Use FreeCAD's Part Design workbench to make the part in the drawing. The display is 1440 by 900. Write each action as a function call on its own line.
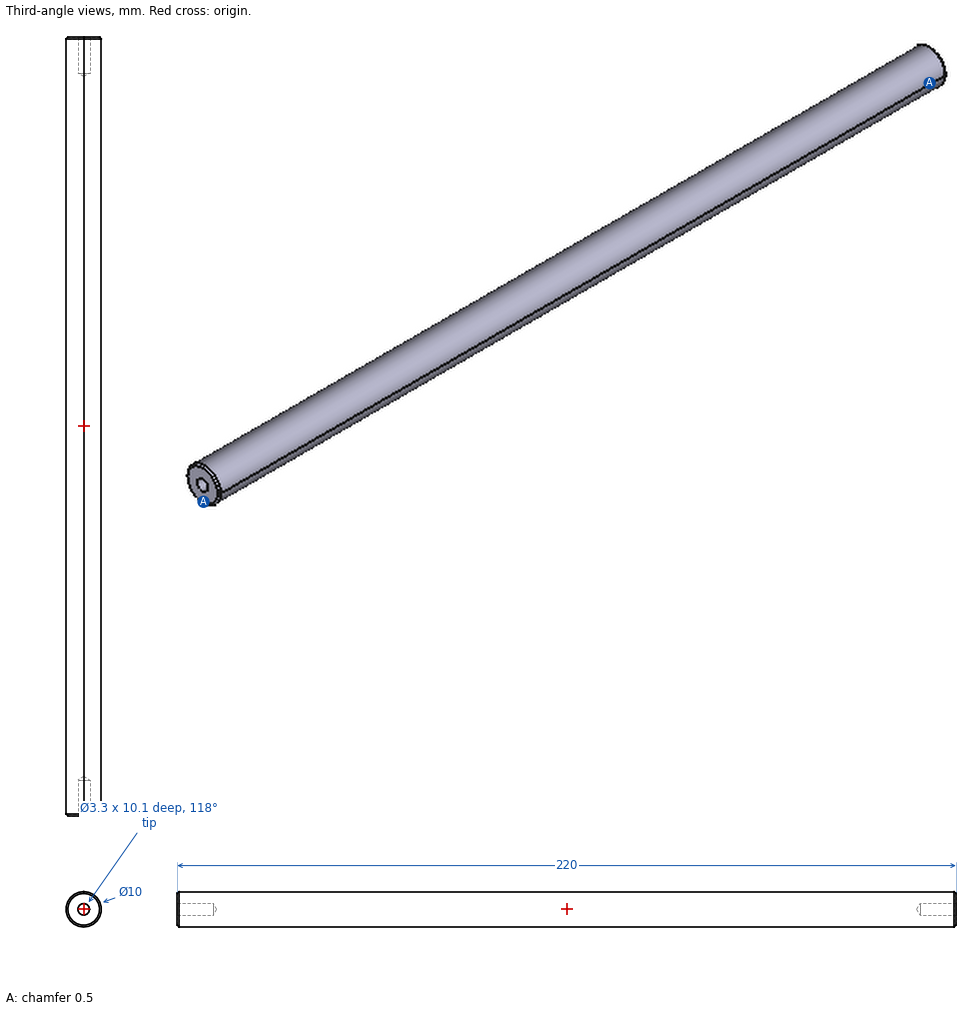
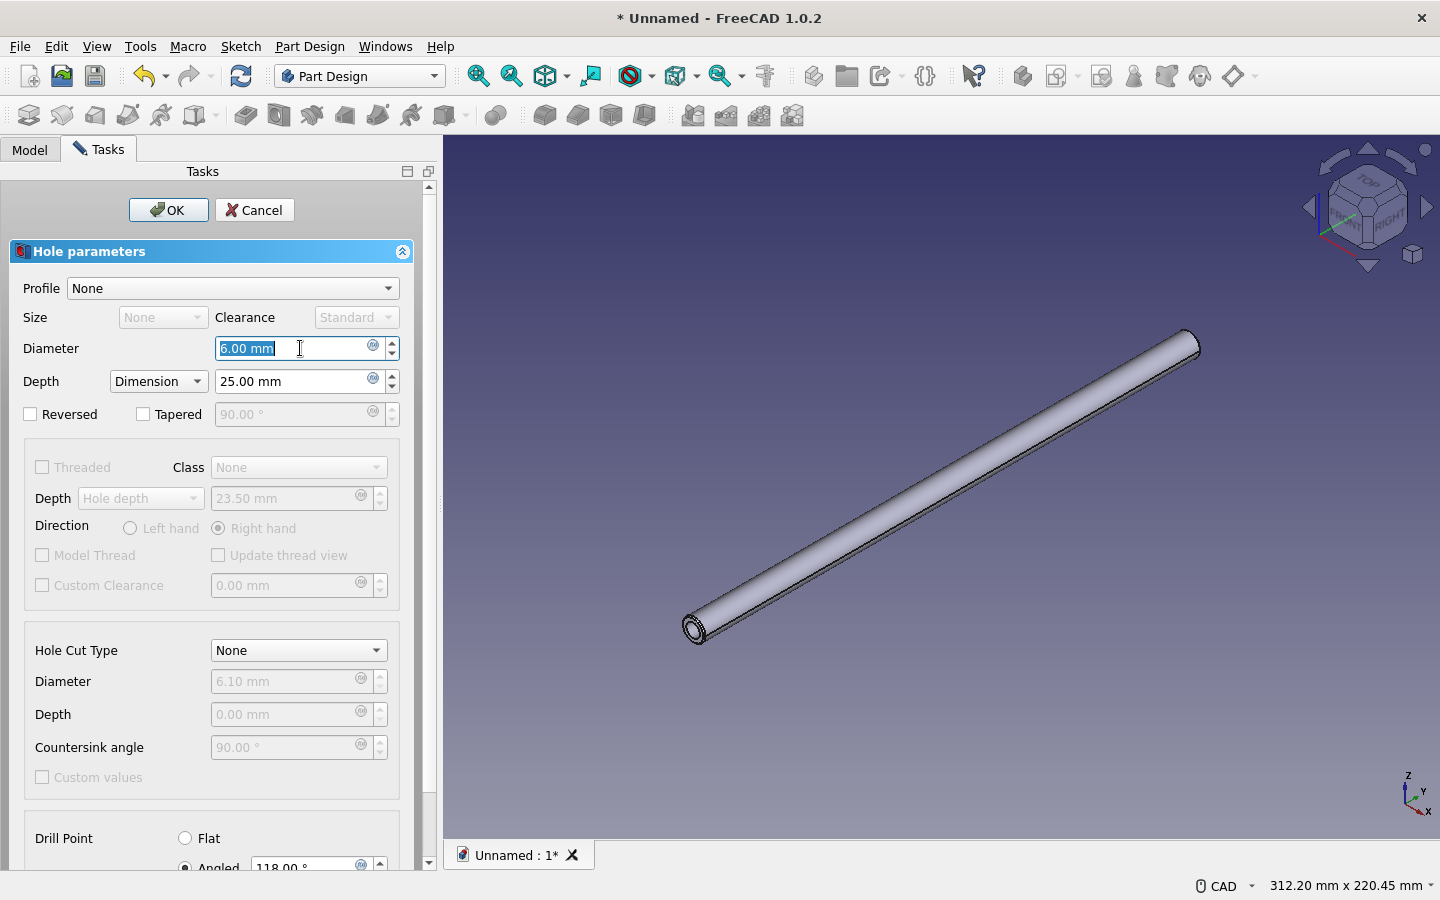
text(3.3)
key(Tab)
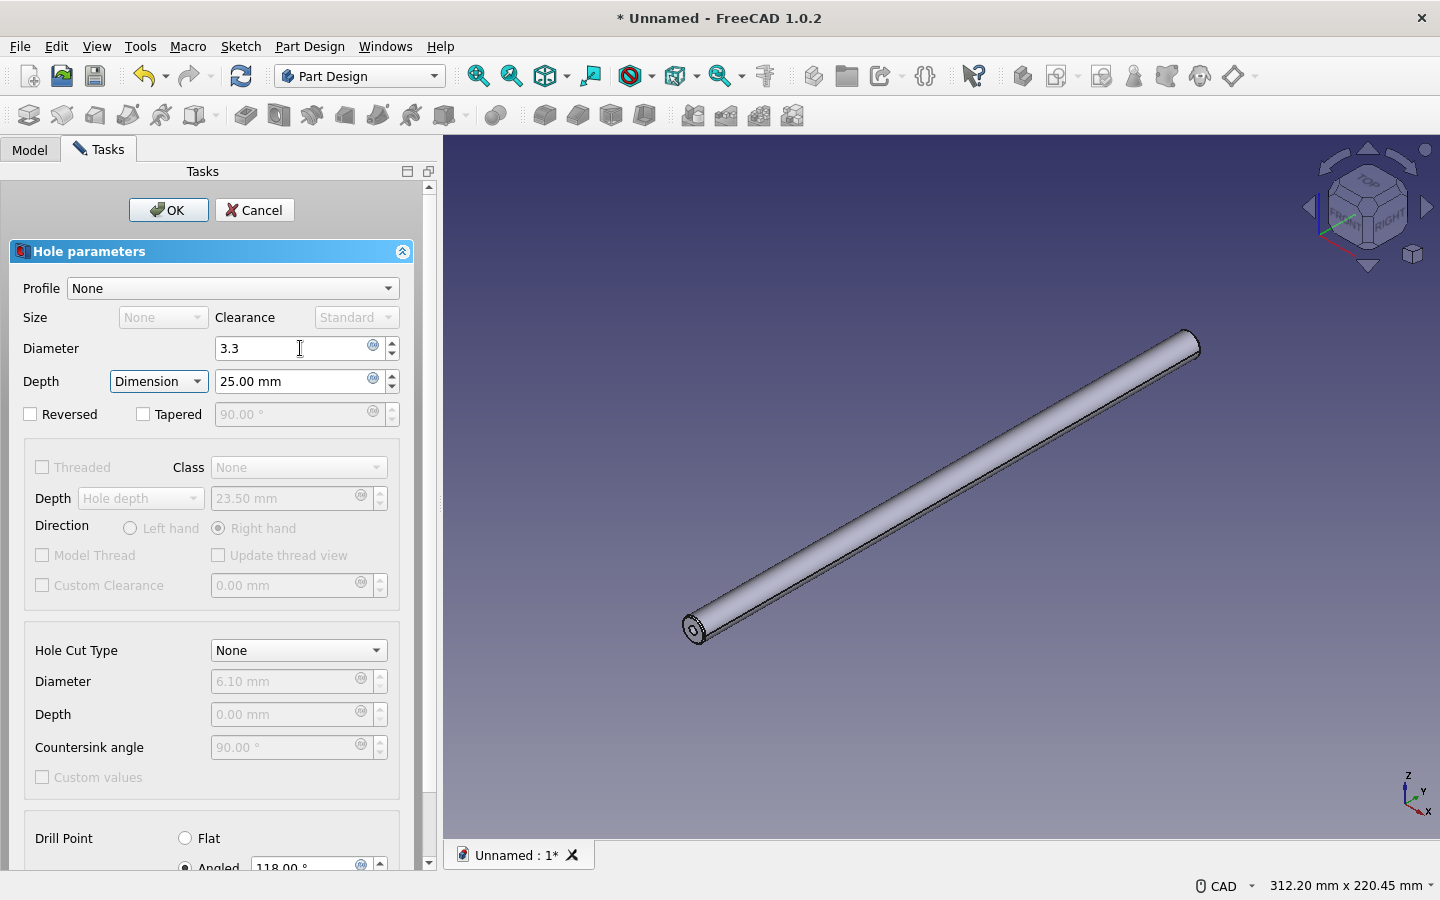
triple_click(300, 382)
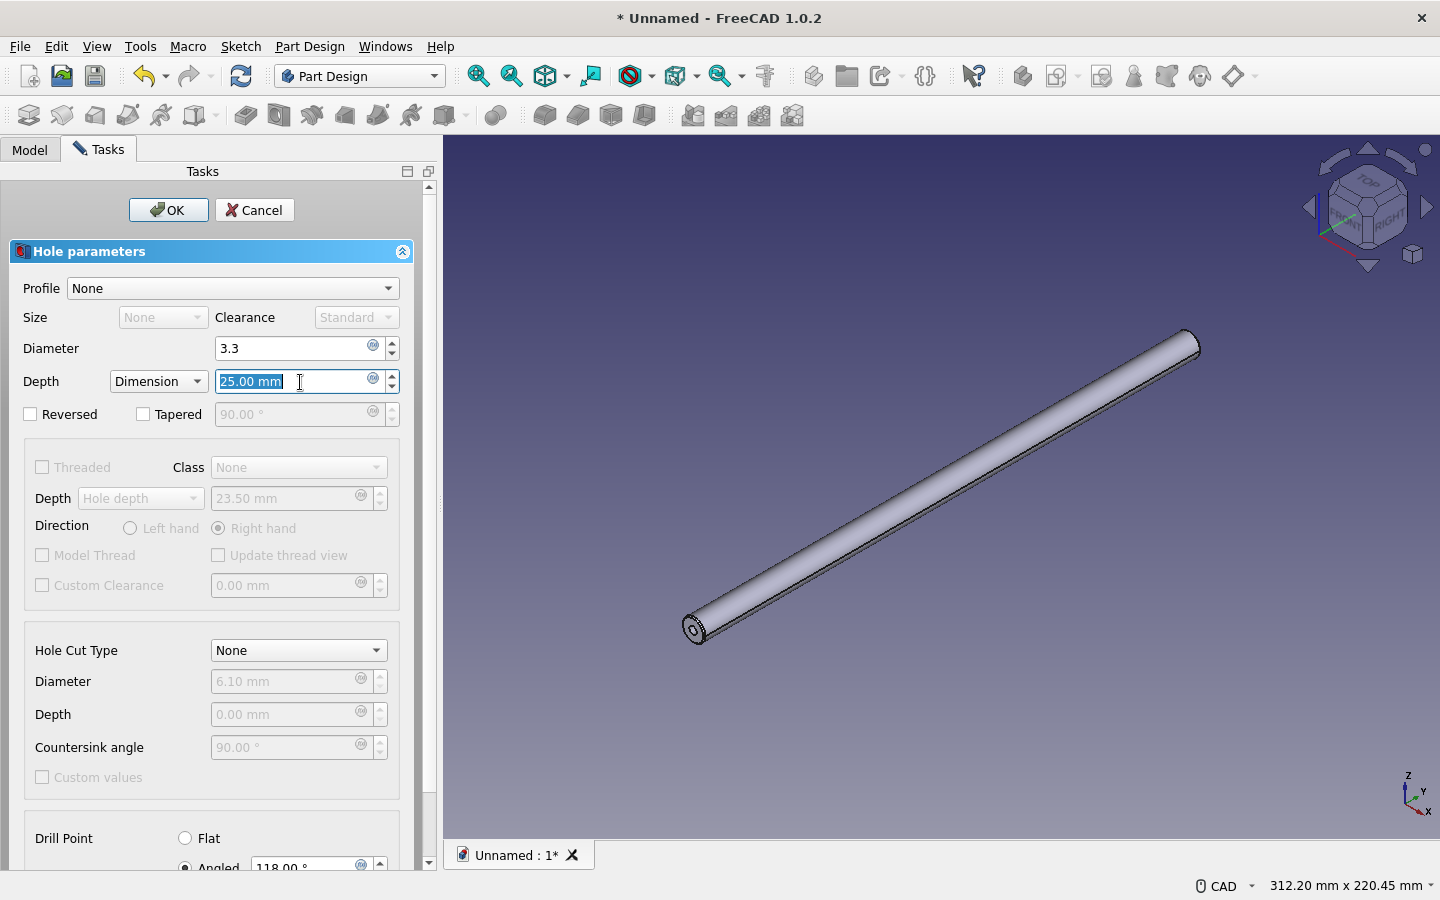
text(10.1)
key(Tab)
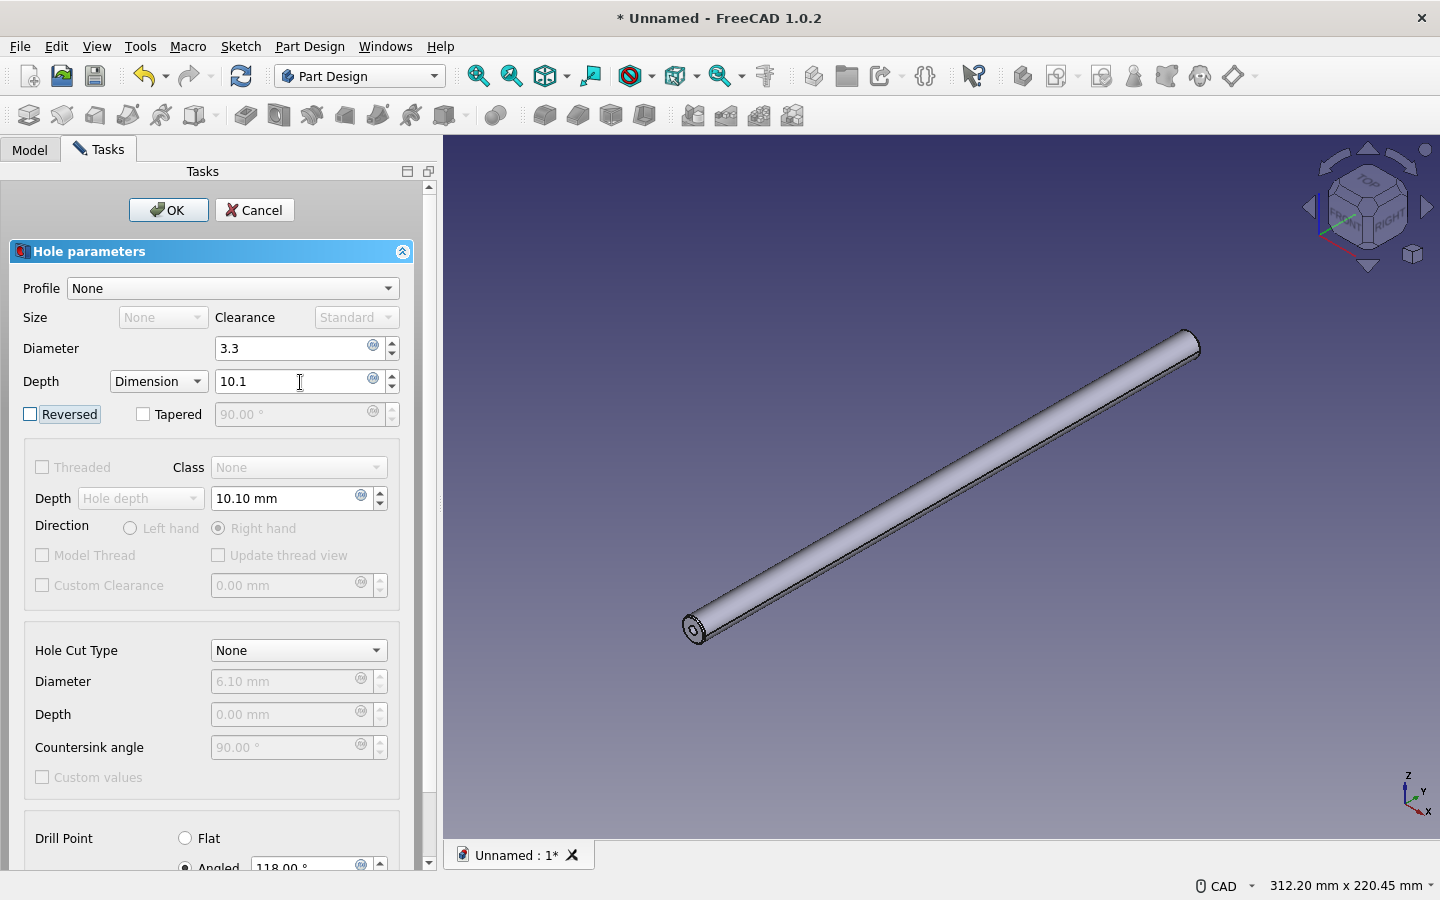
click(169, 210)